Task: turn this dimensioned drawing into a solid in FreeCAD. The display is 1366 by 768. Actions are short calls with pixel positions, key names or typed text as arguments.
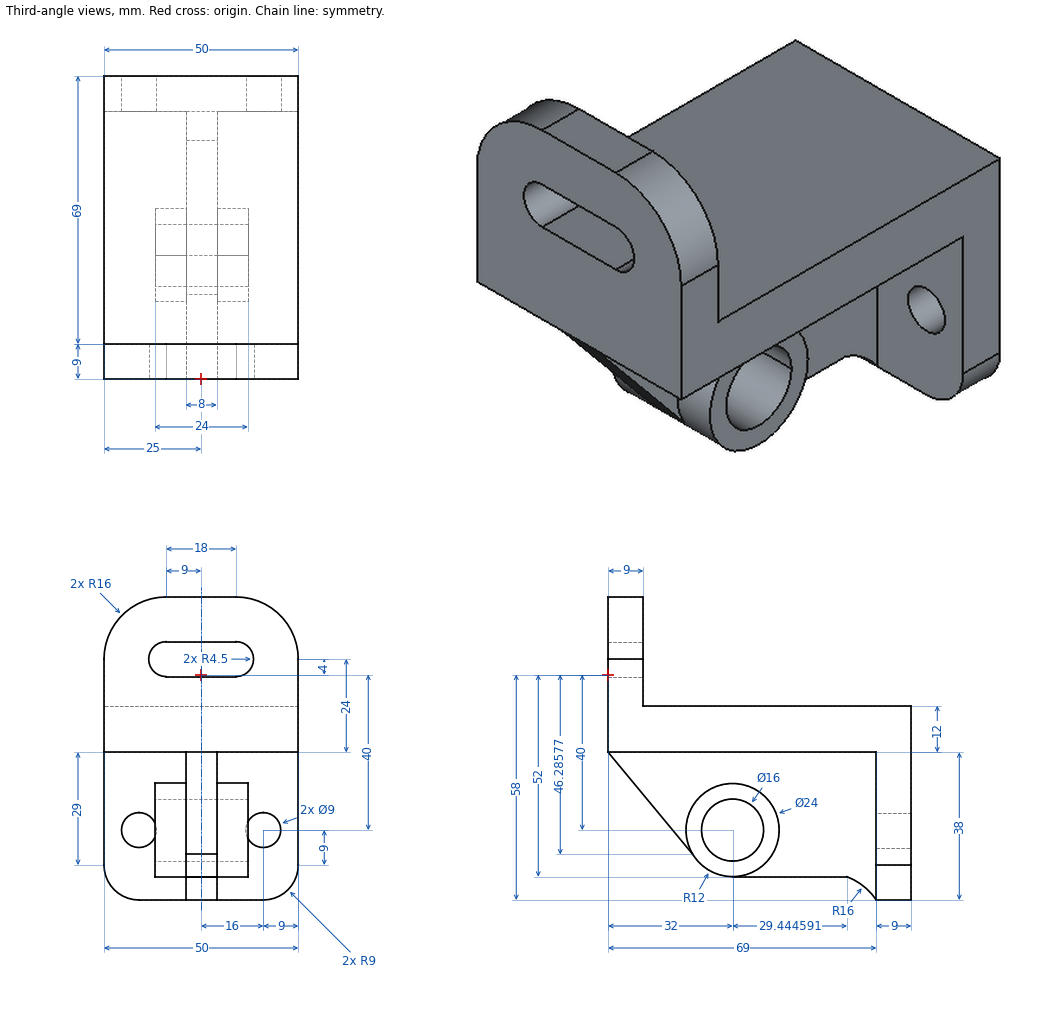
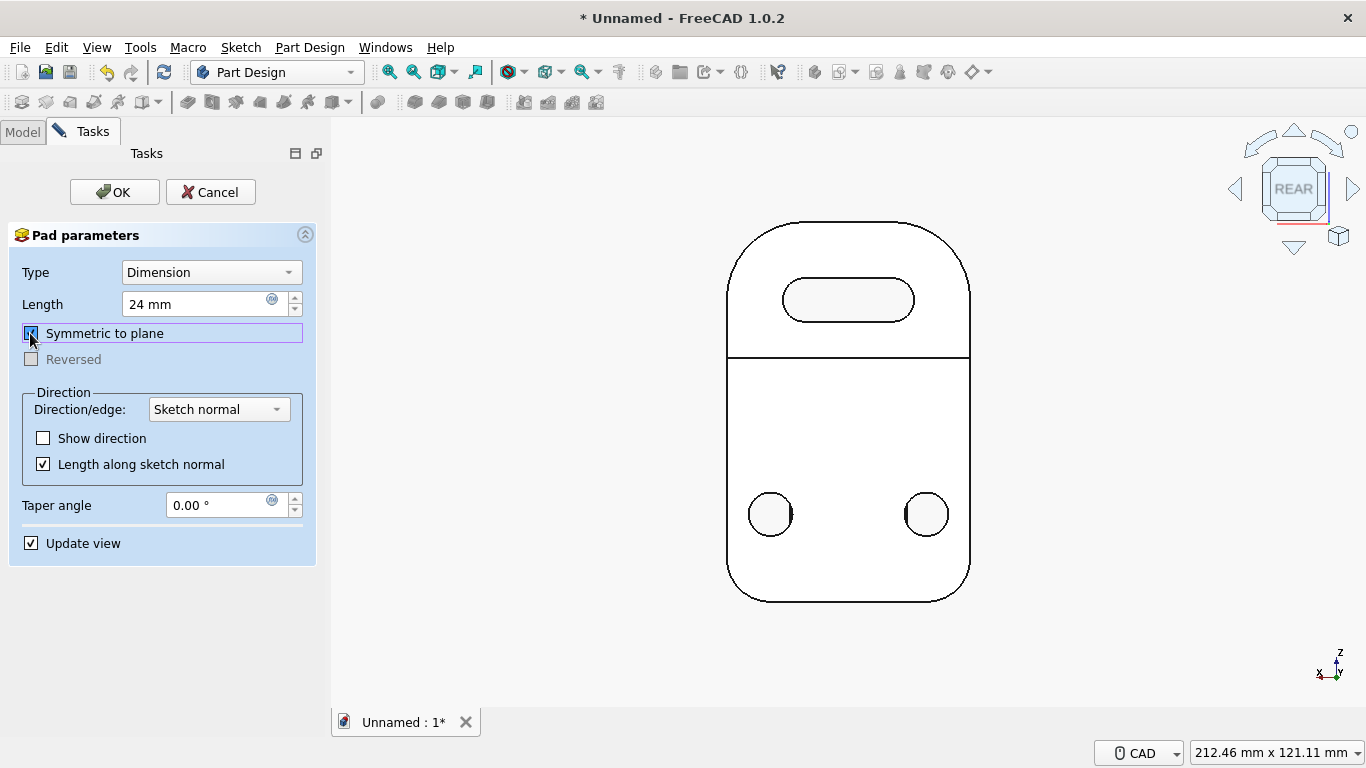
click(115, 192)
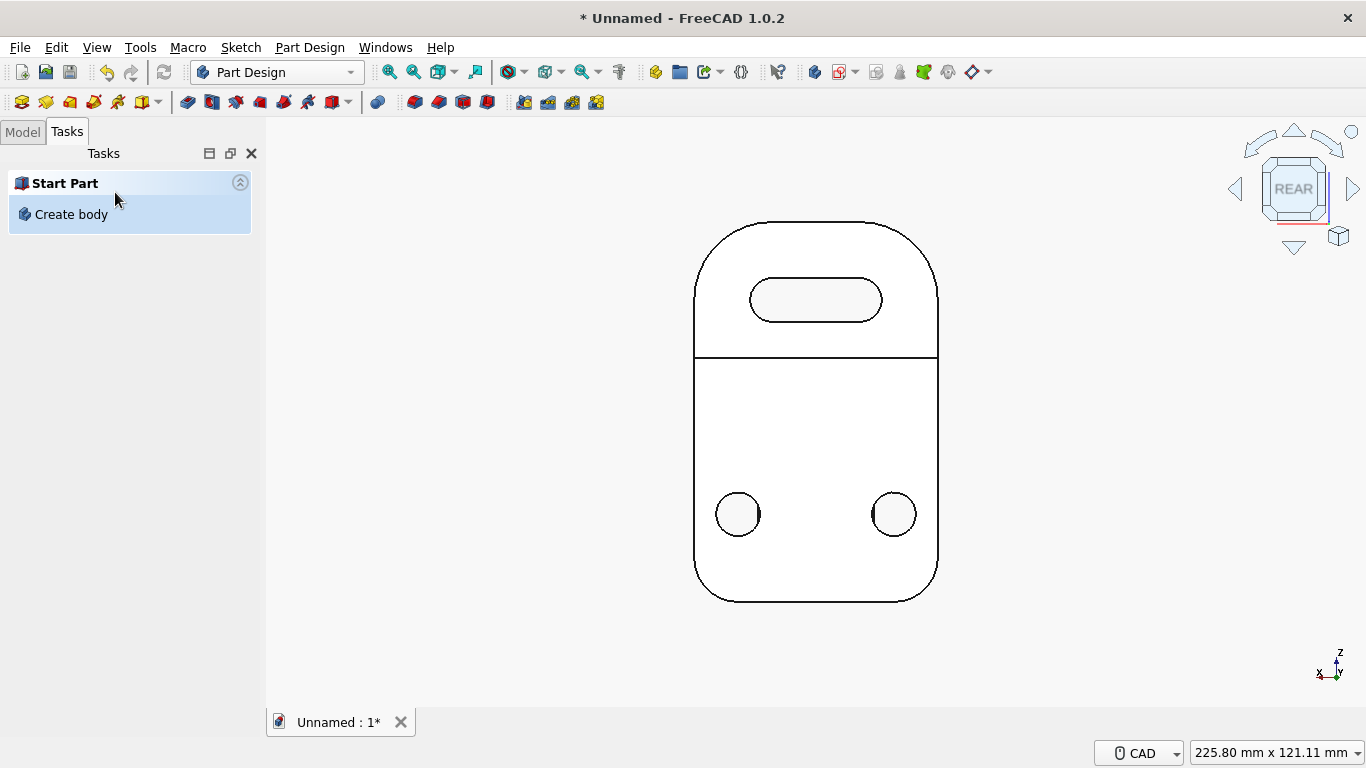
click(390, 72)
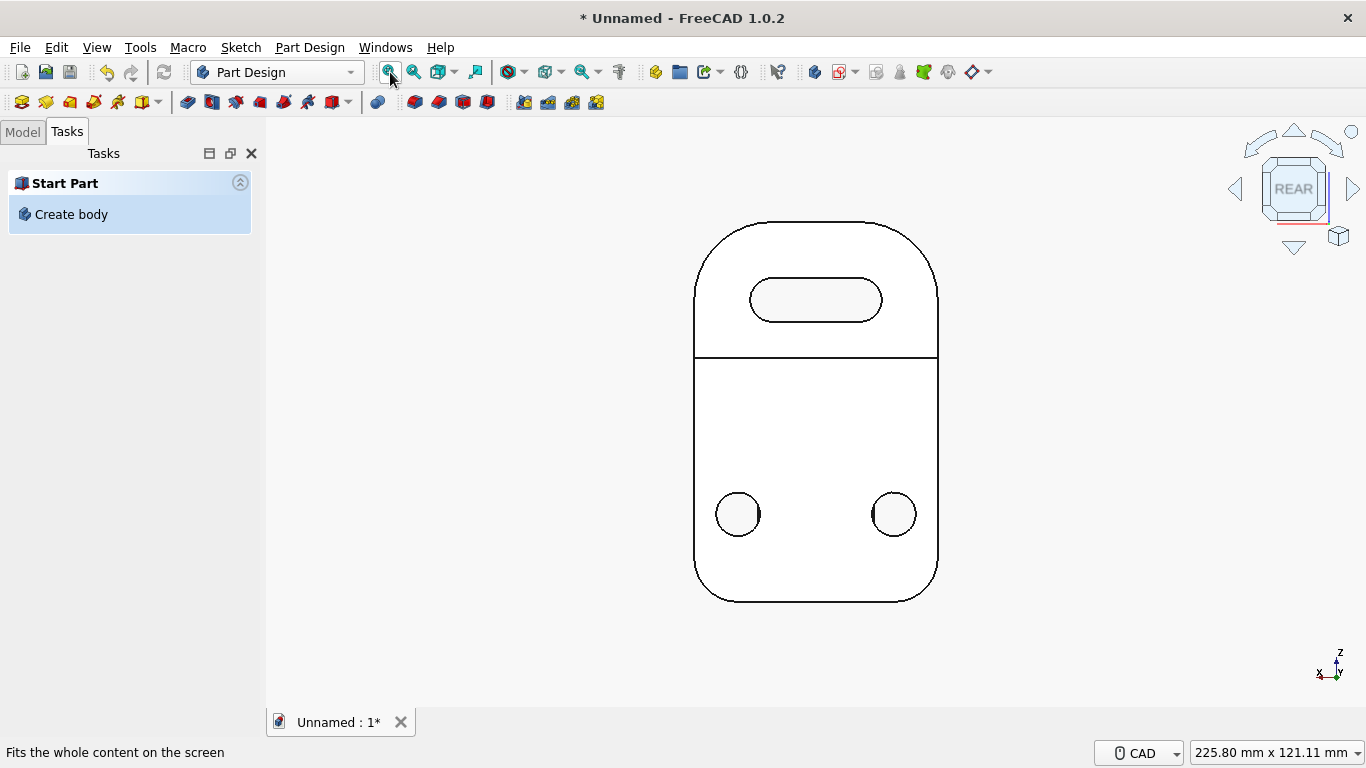
click(23, 131)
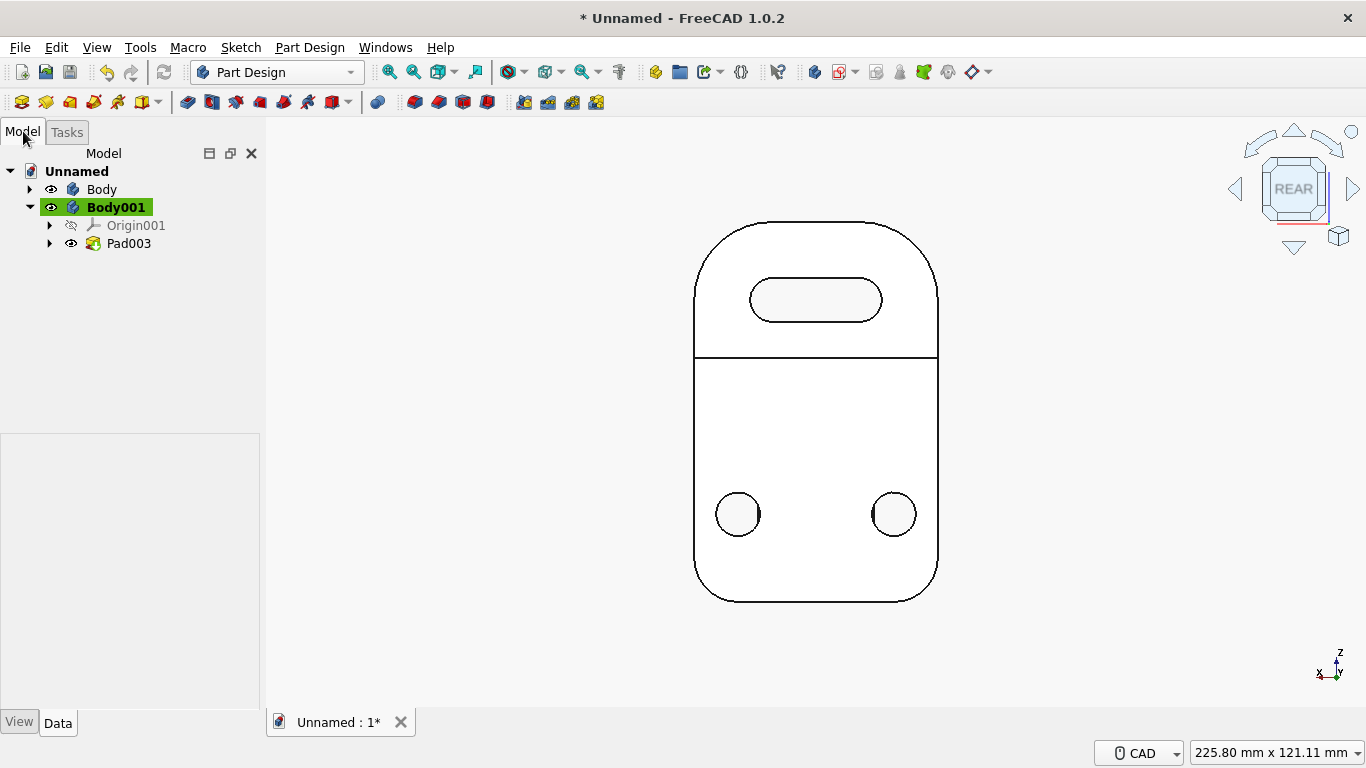
double_click(96, 189)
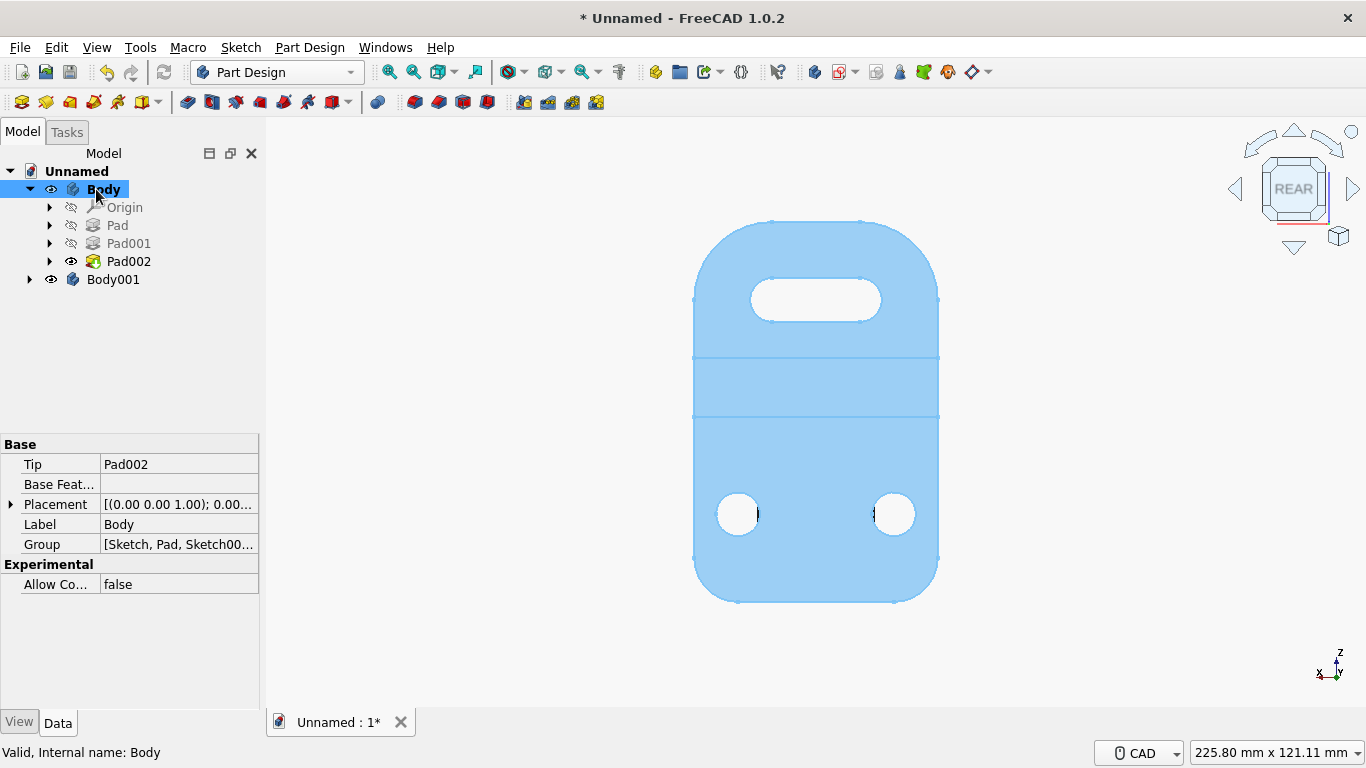
click(96, 189)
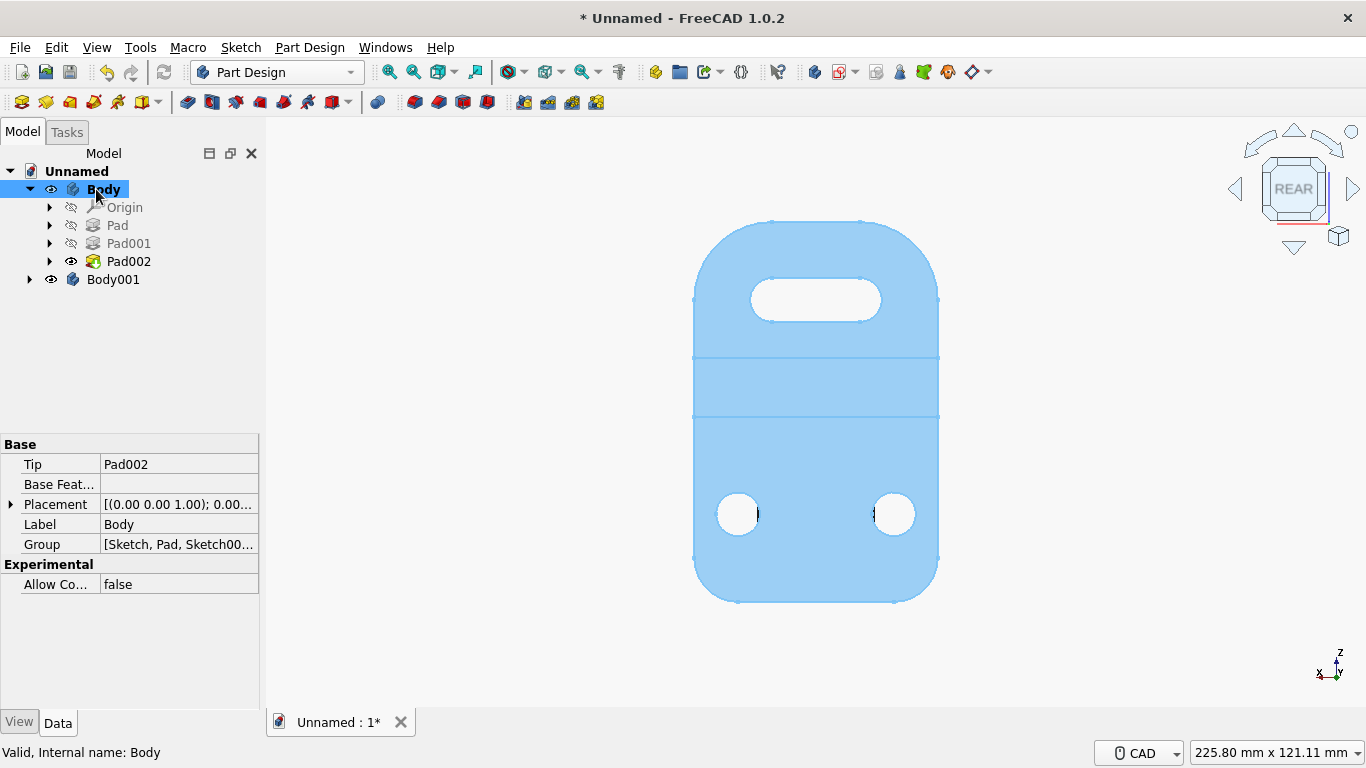
click(146, 584)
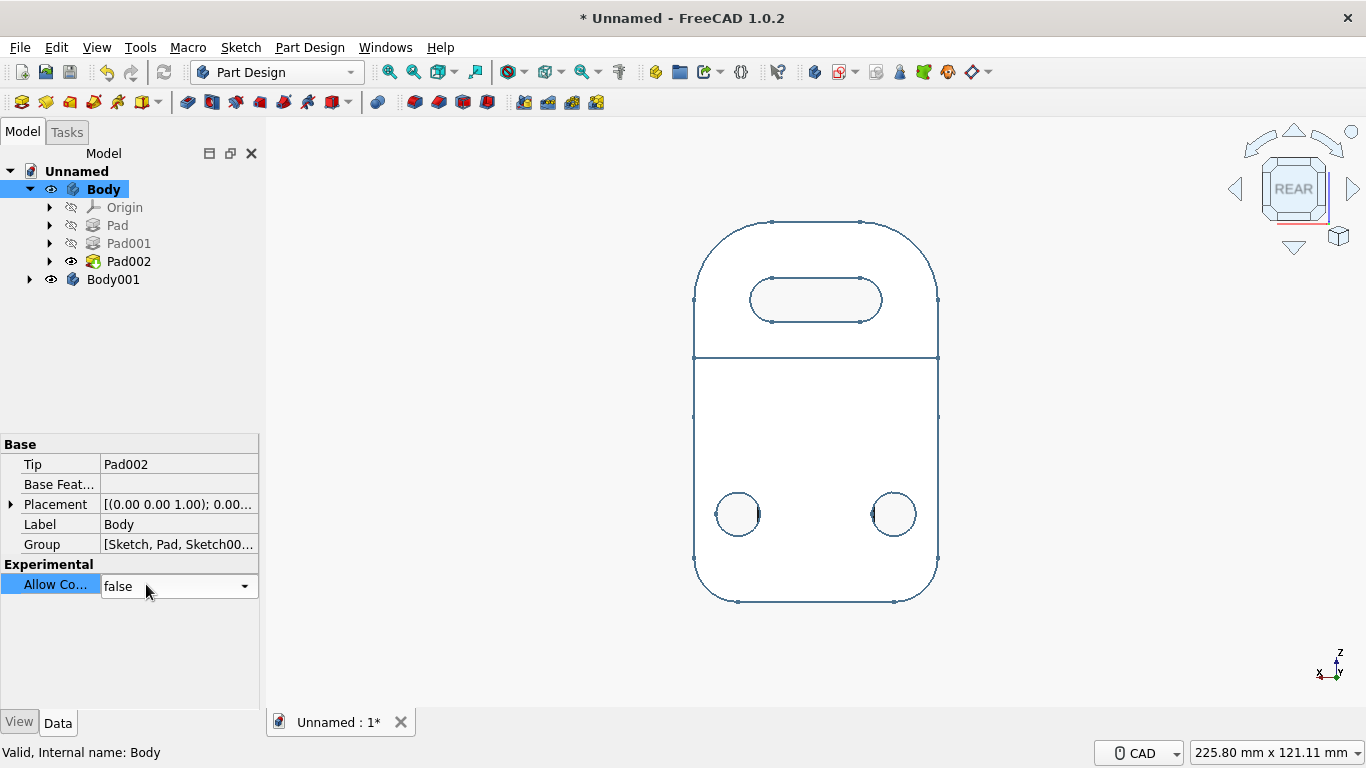
click(146, 584)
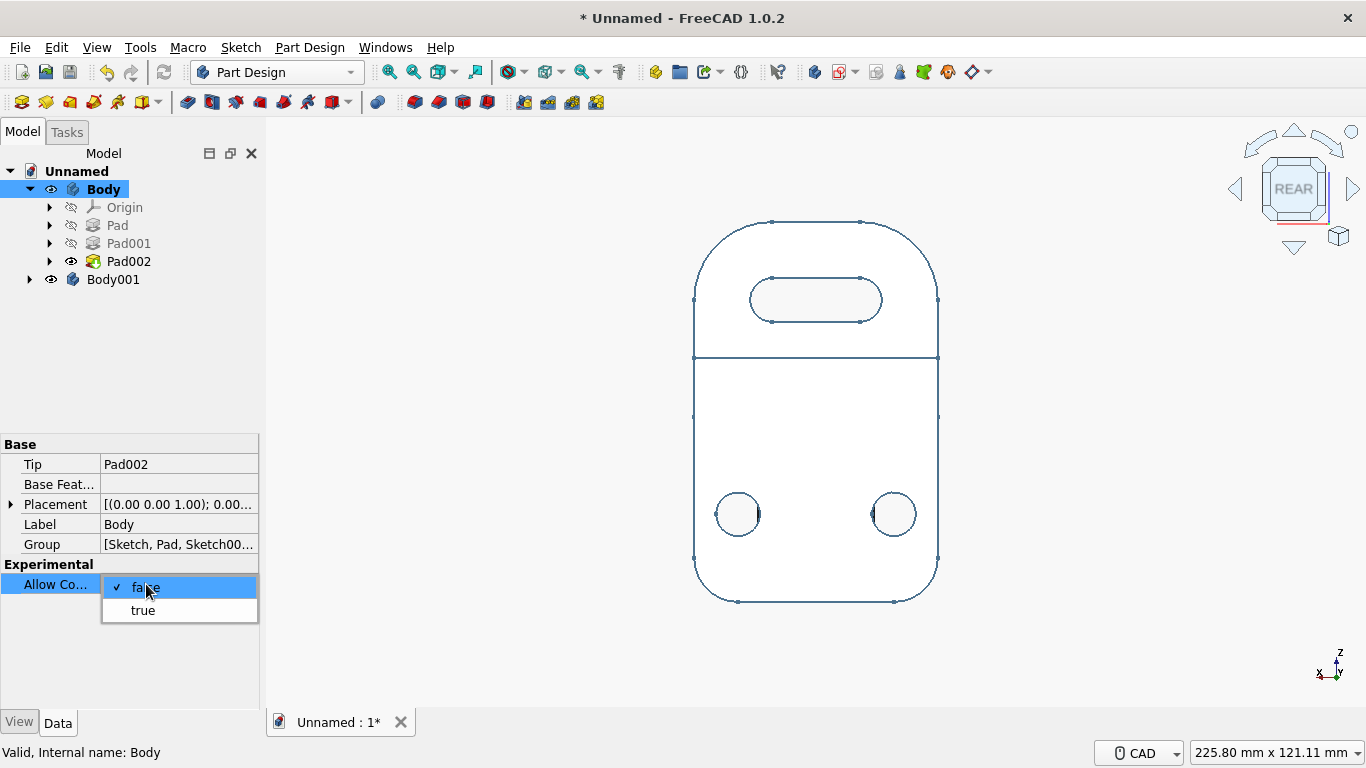
click(179, 610)
key(Return)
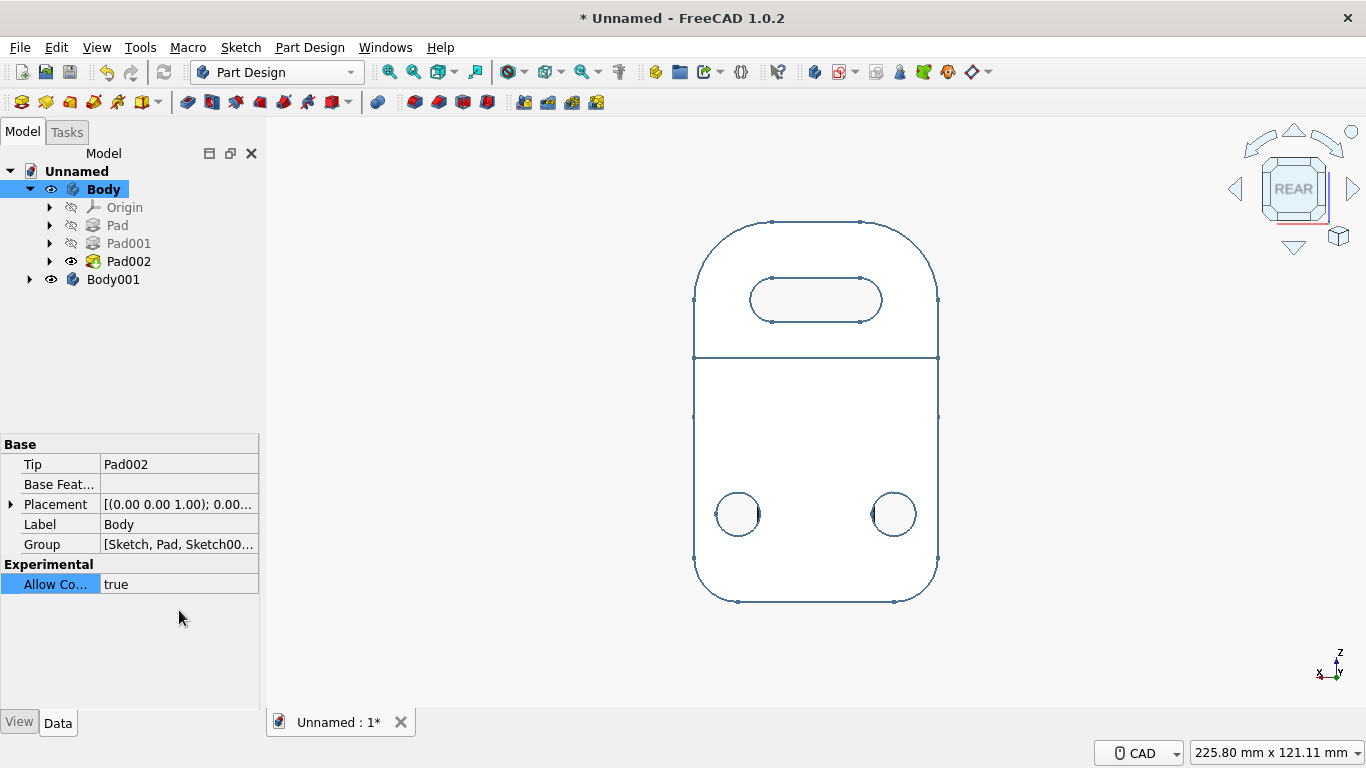
click(96, 279)